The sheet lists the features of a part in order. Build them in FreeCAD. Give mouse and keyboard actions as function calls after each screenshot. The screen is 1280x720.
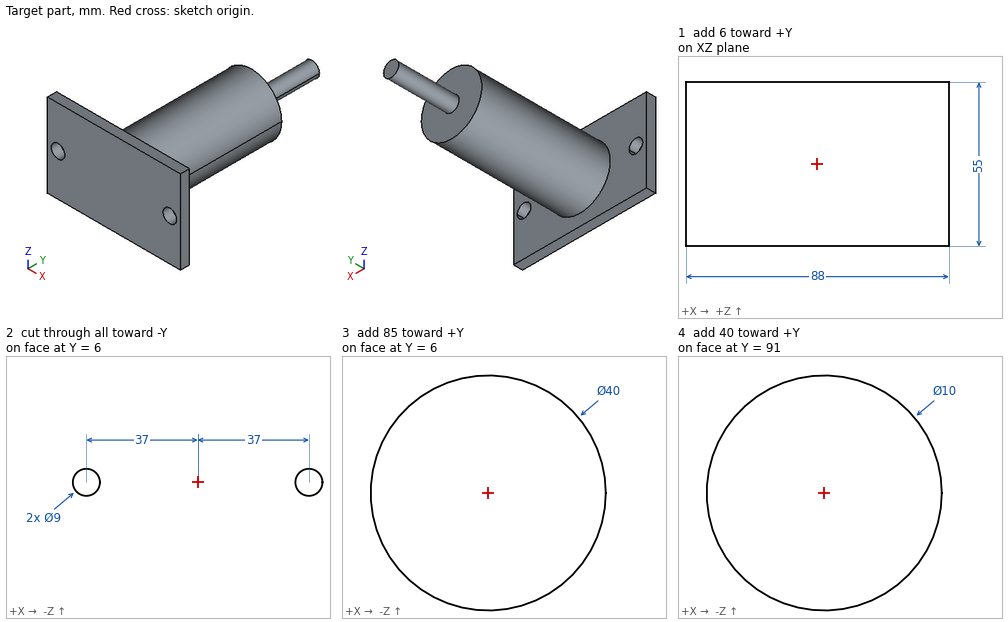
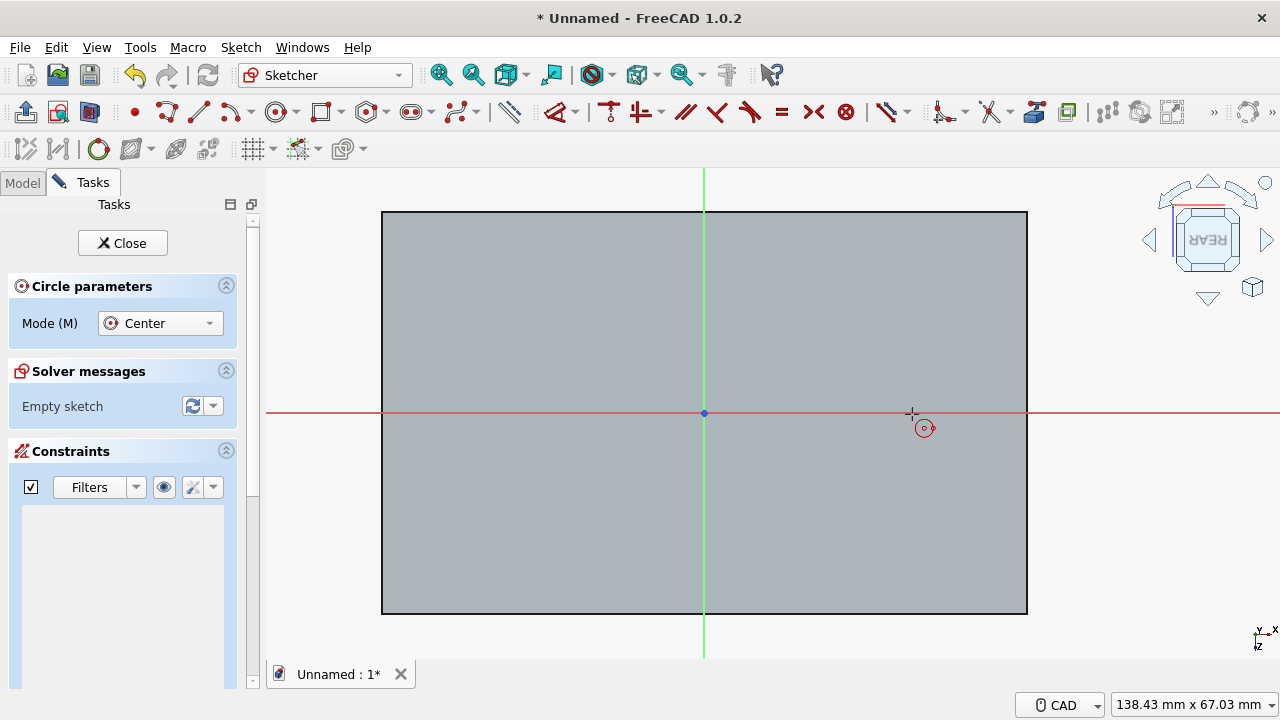
click(433, 413)
click(457, 390)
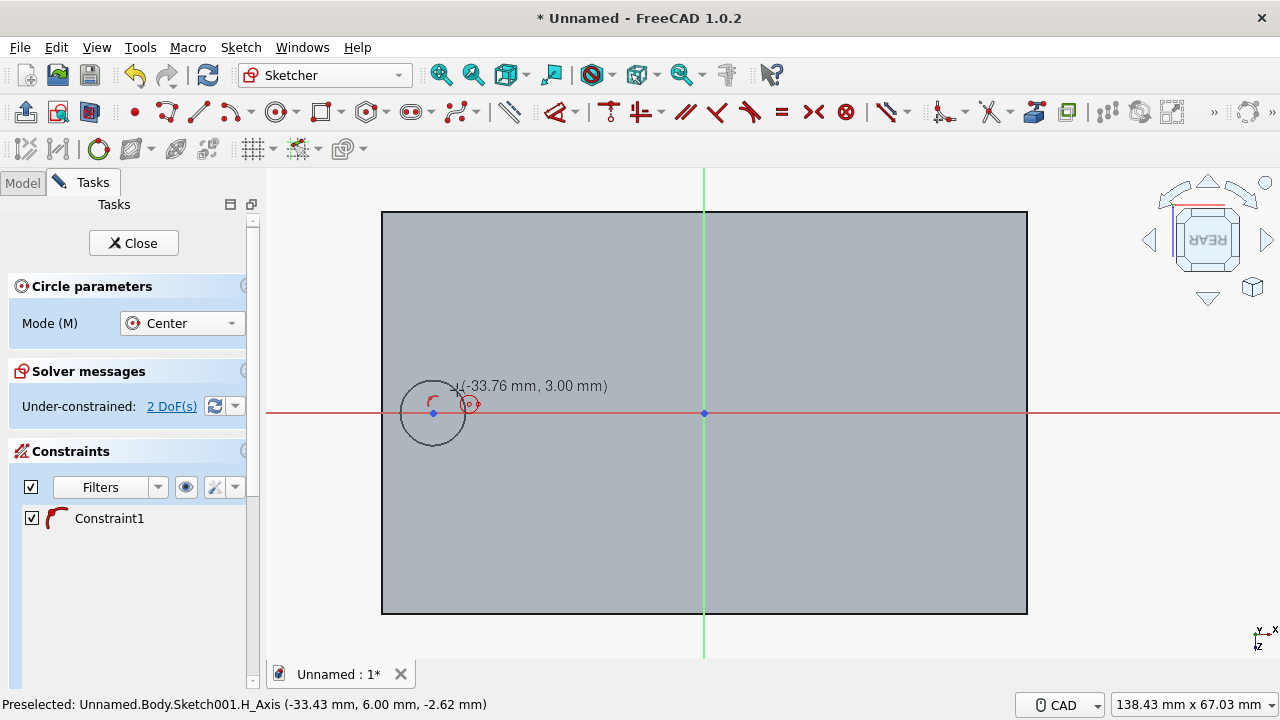
click(975, 413)
click(999, 390)
key(Escape)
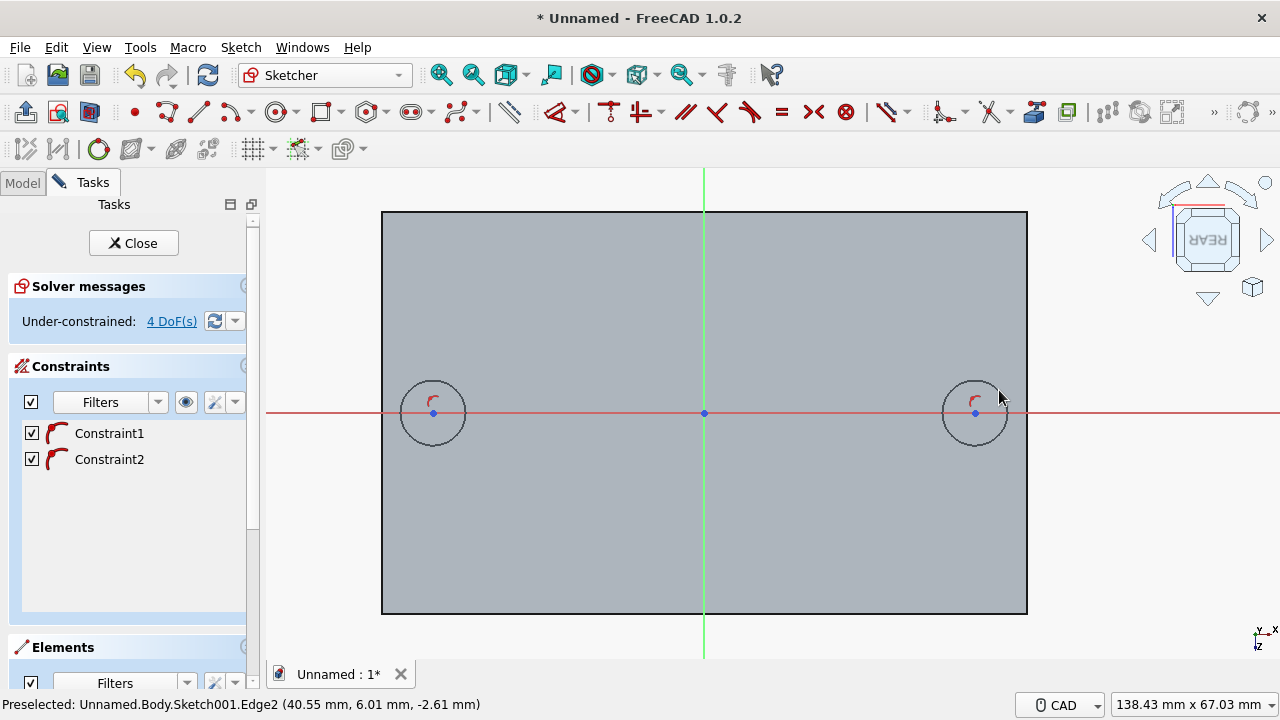
click(456, 390)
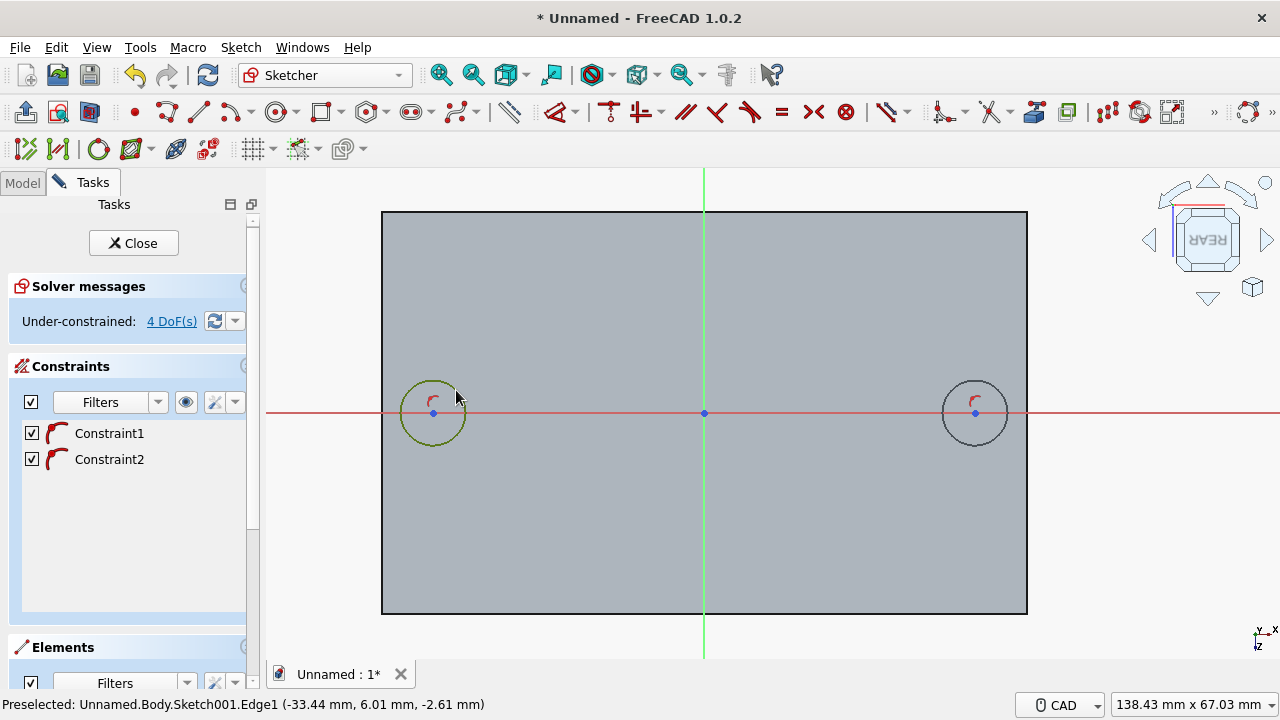
click(998, 390)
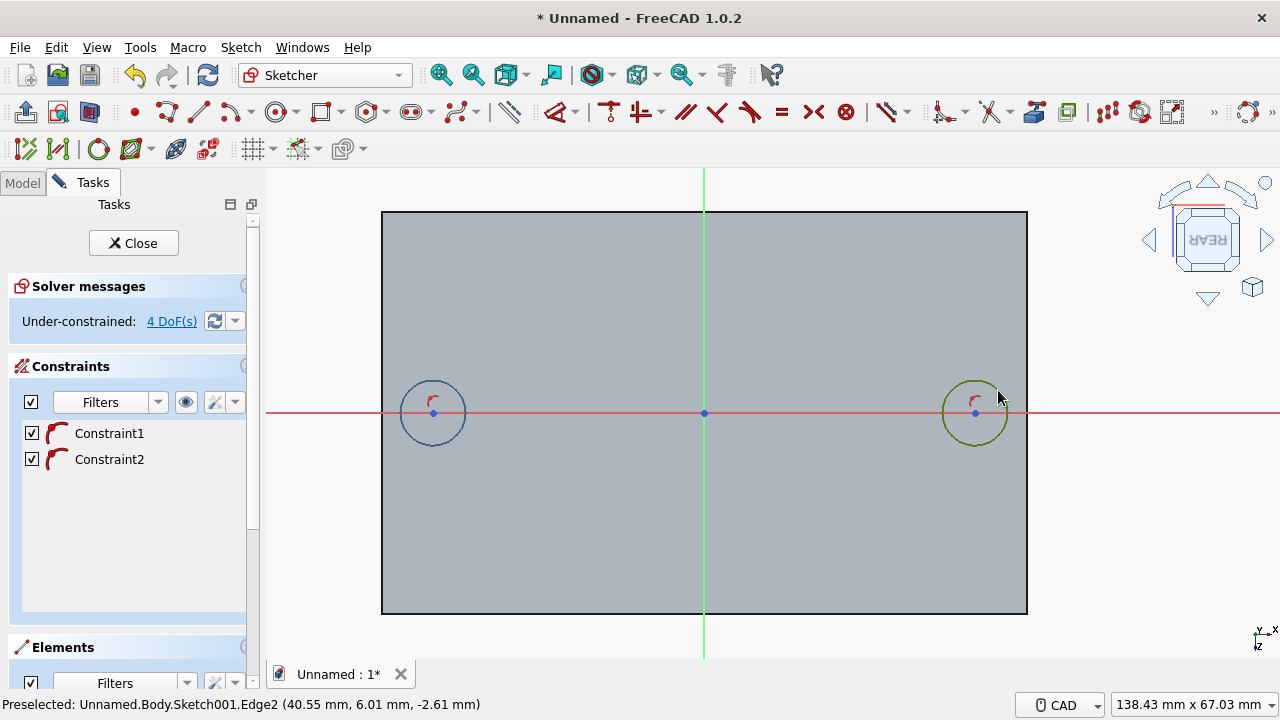
key(e)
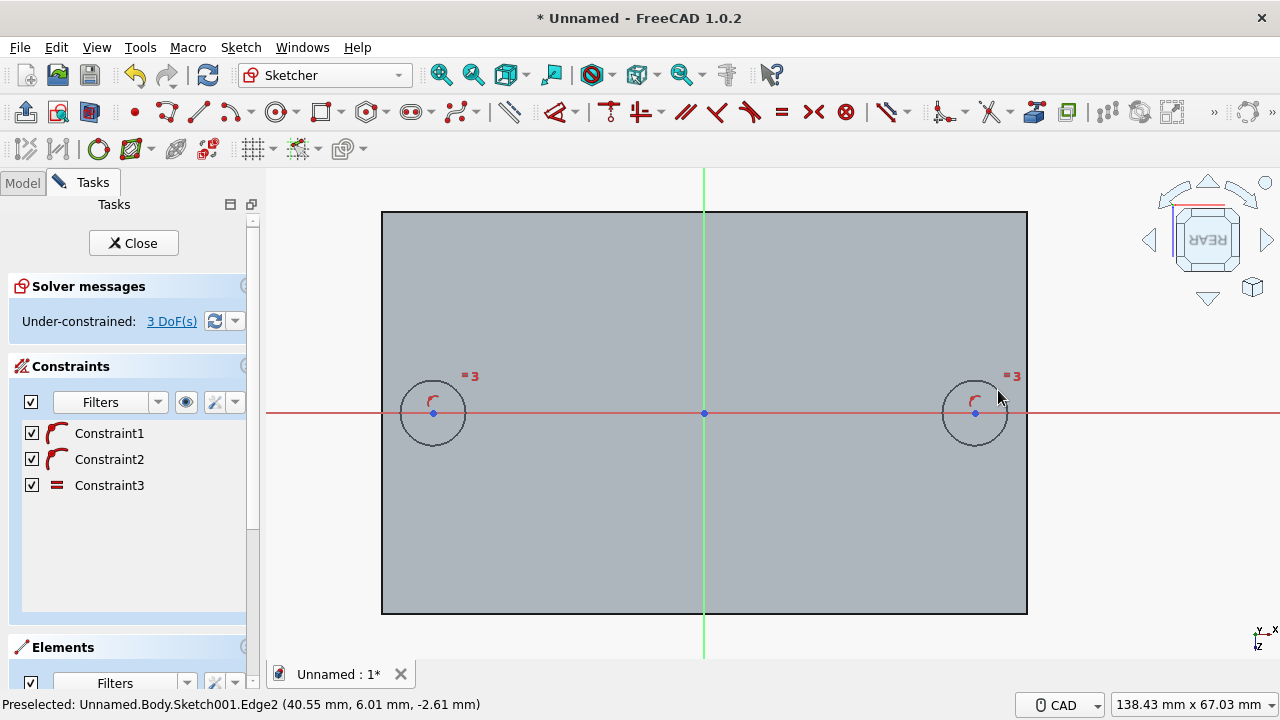
click(456, 390)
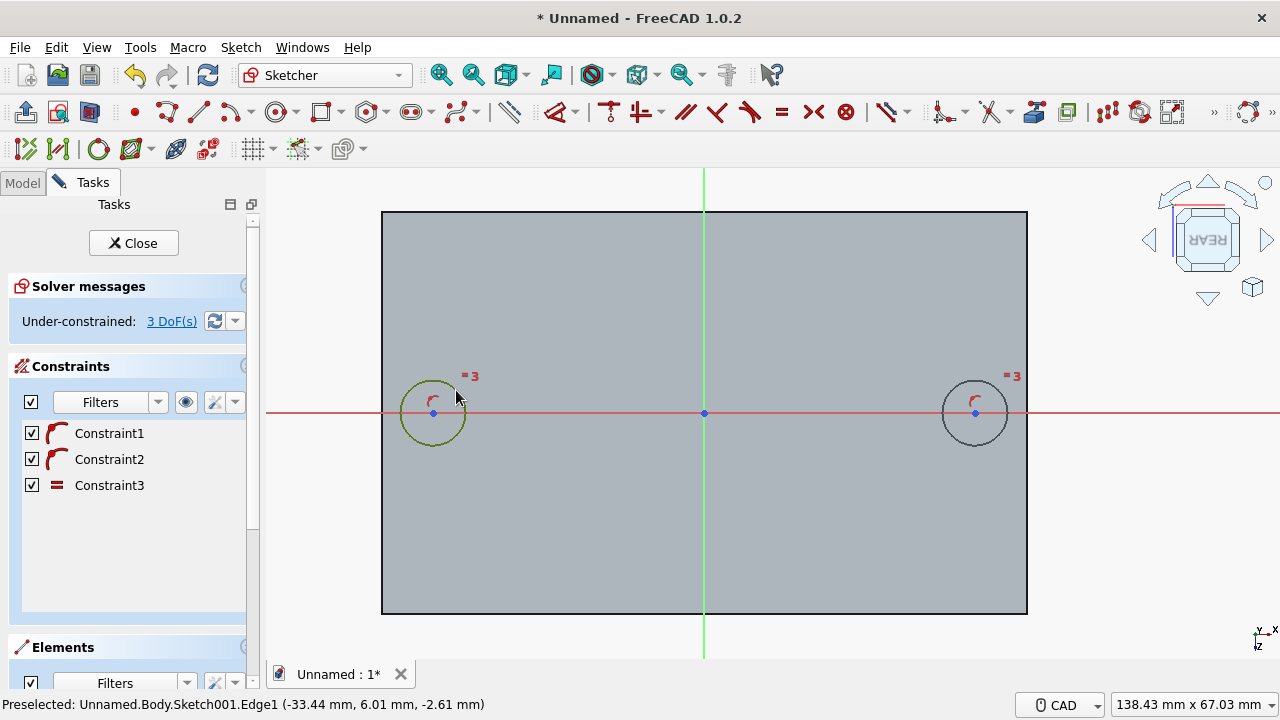
key(k)
key(o)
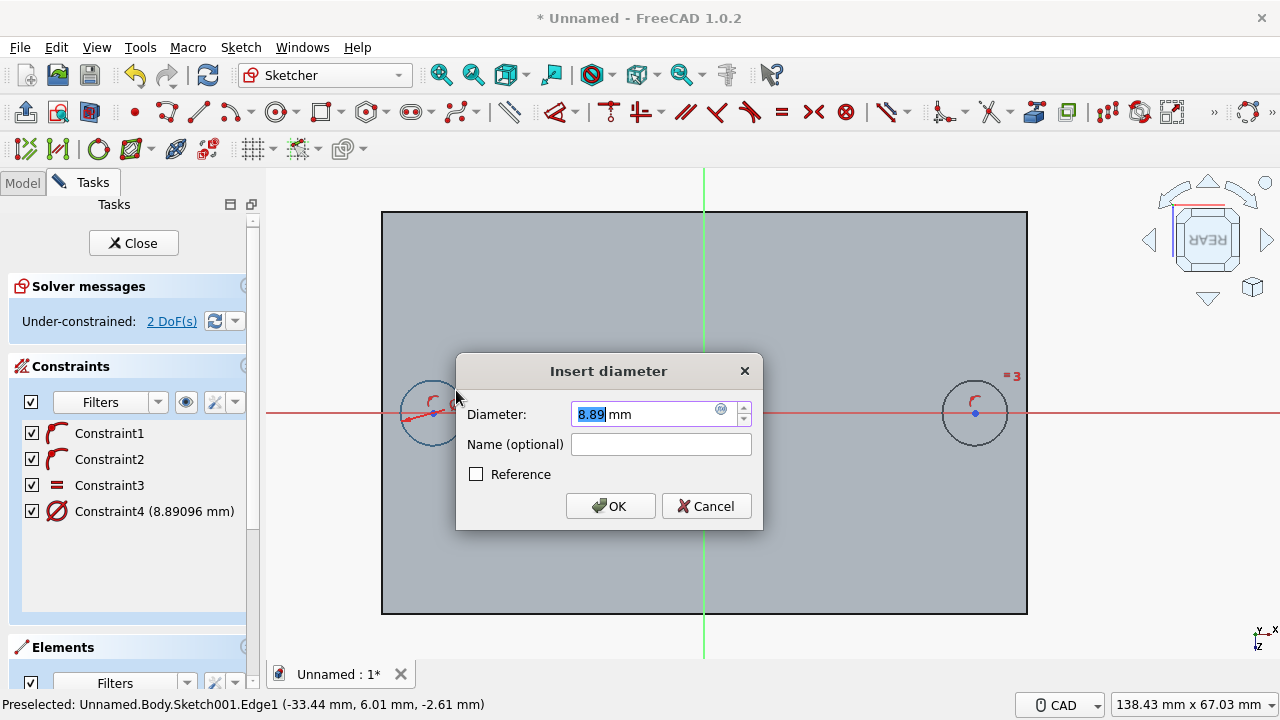
text(9)
key(Return)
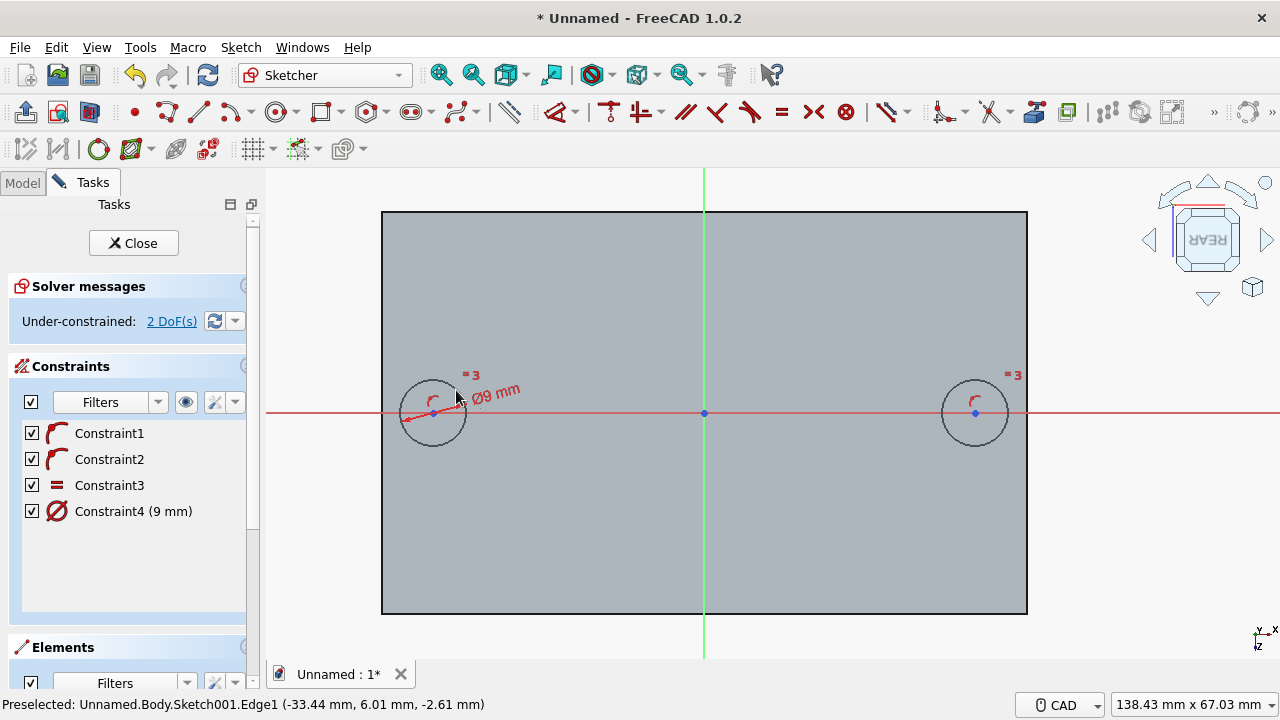
click(433, 413)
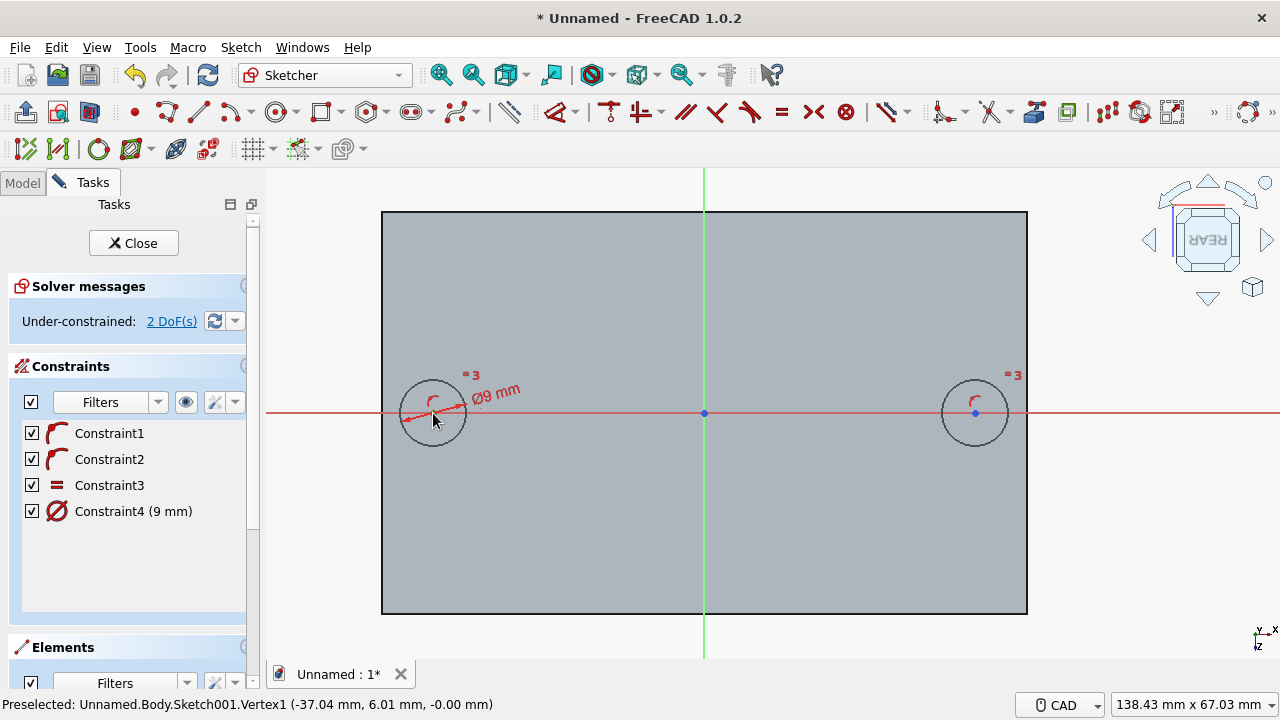
key(l)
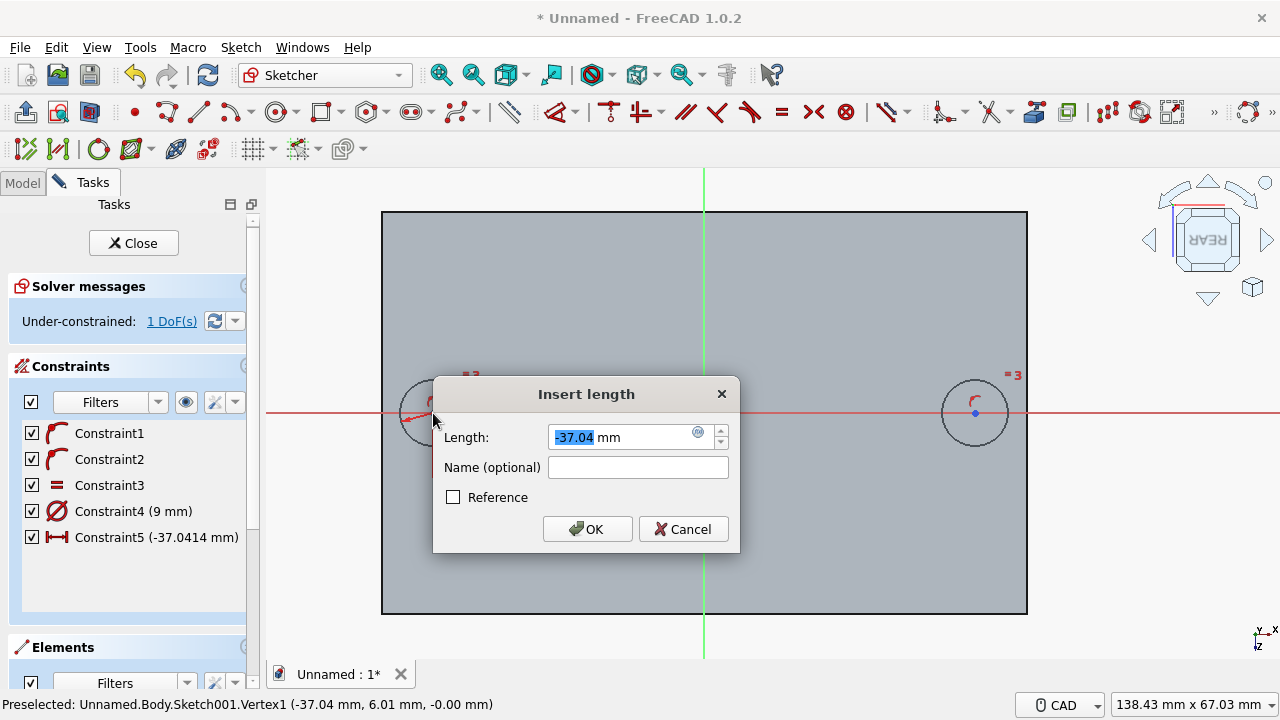
text(-37)
key(Return)